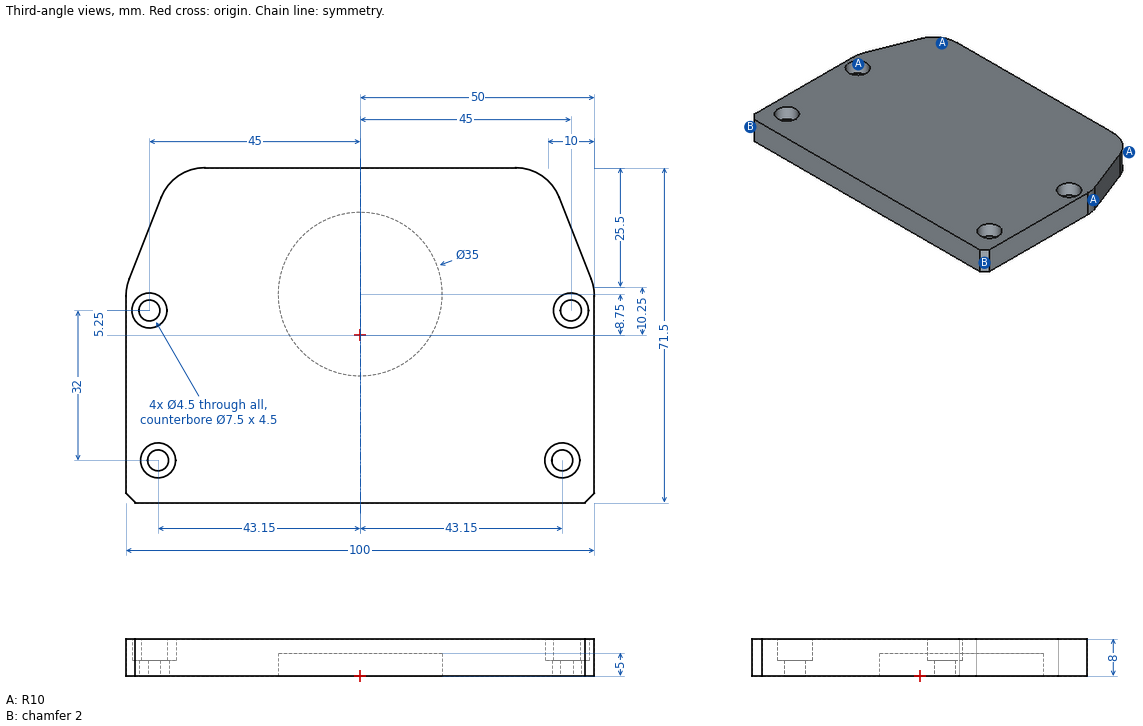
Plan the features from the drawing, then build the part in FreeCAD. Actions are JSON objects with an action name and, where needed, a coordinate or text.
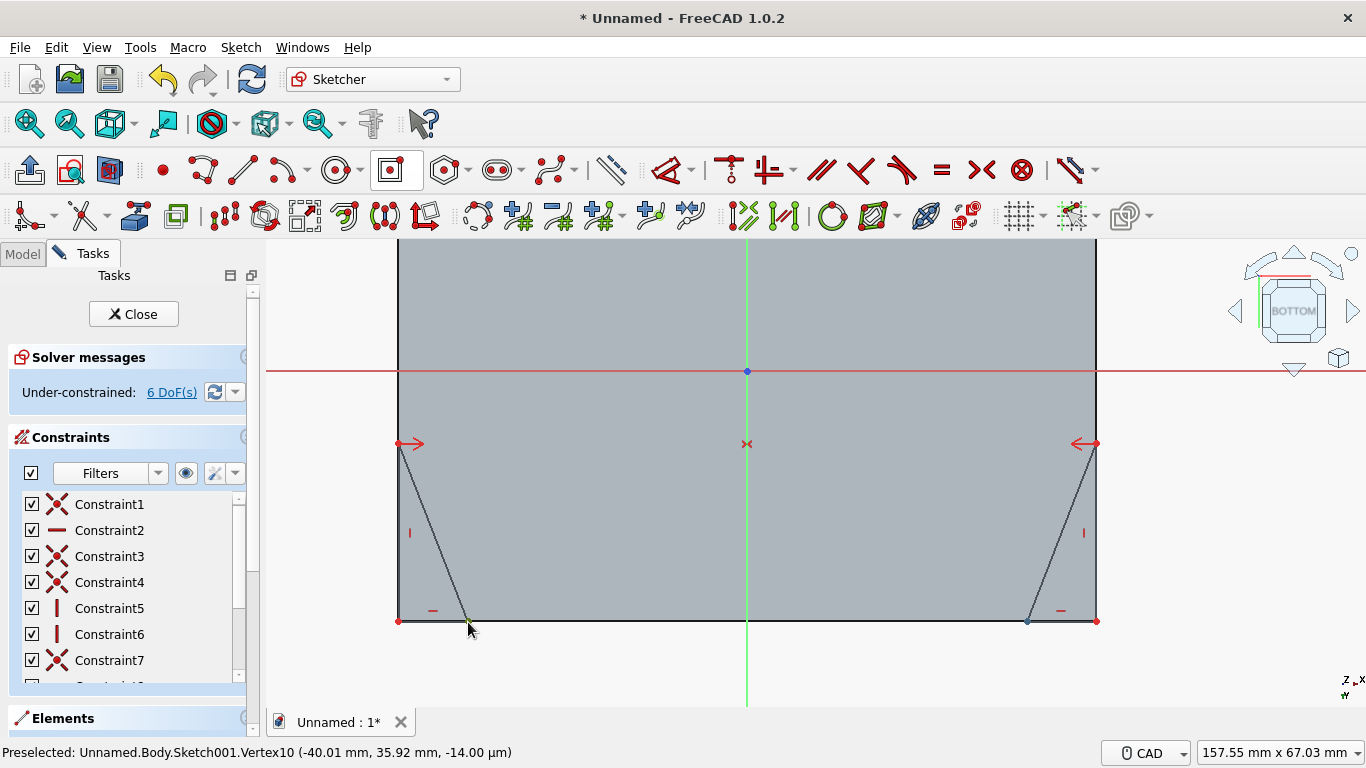
{"action": "left_click", "coordinate": [747, 650]}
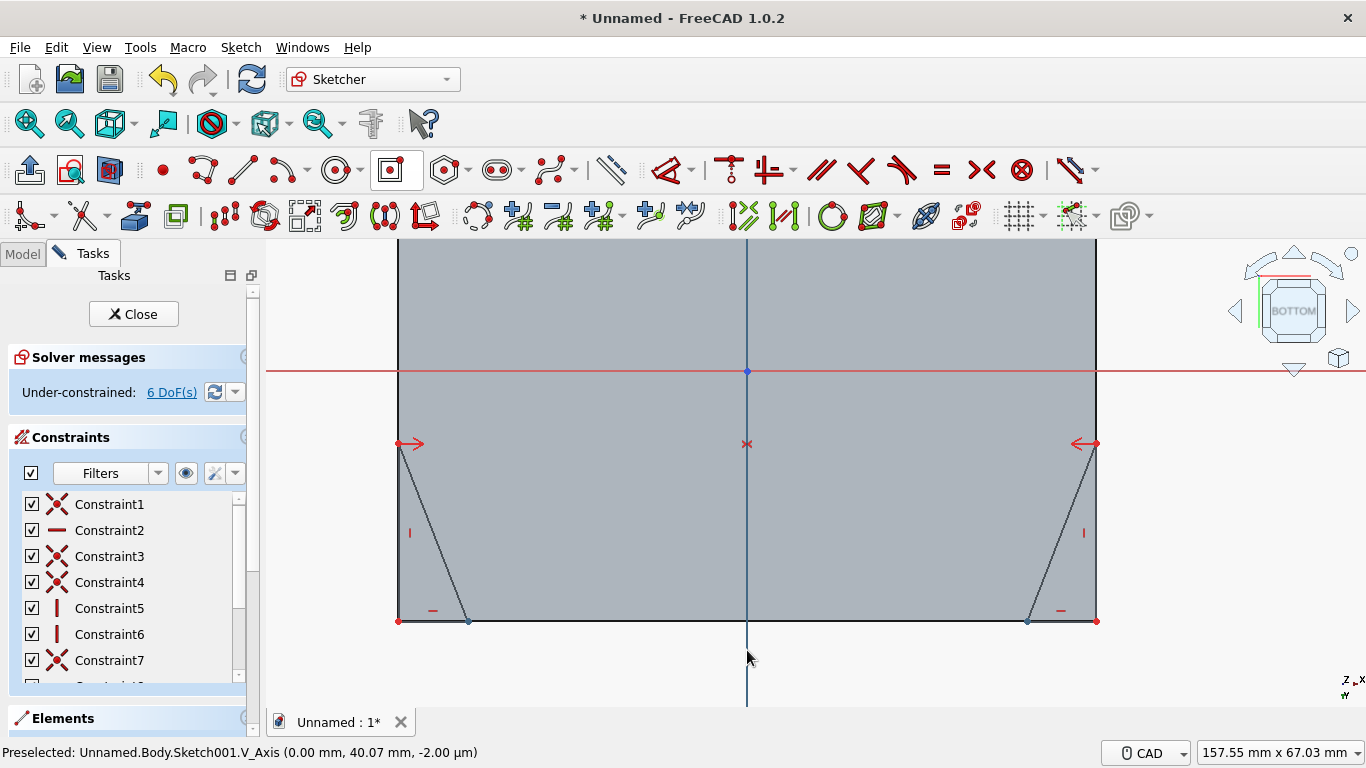
{"action": "left_click", "coordinate": [982, 170]}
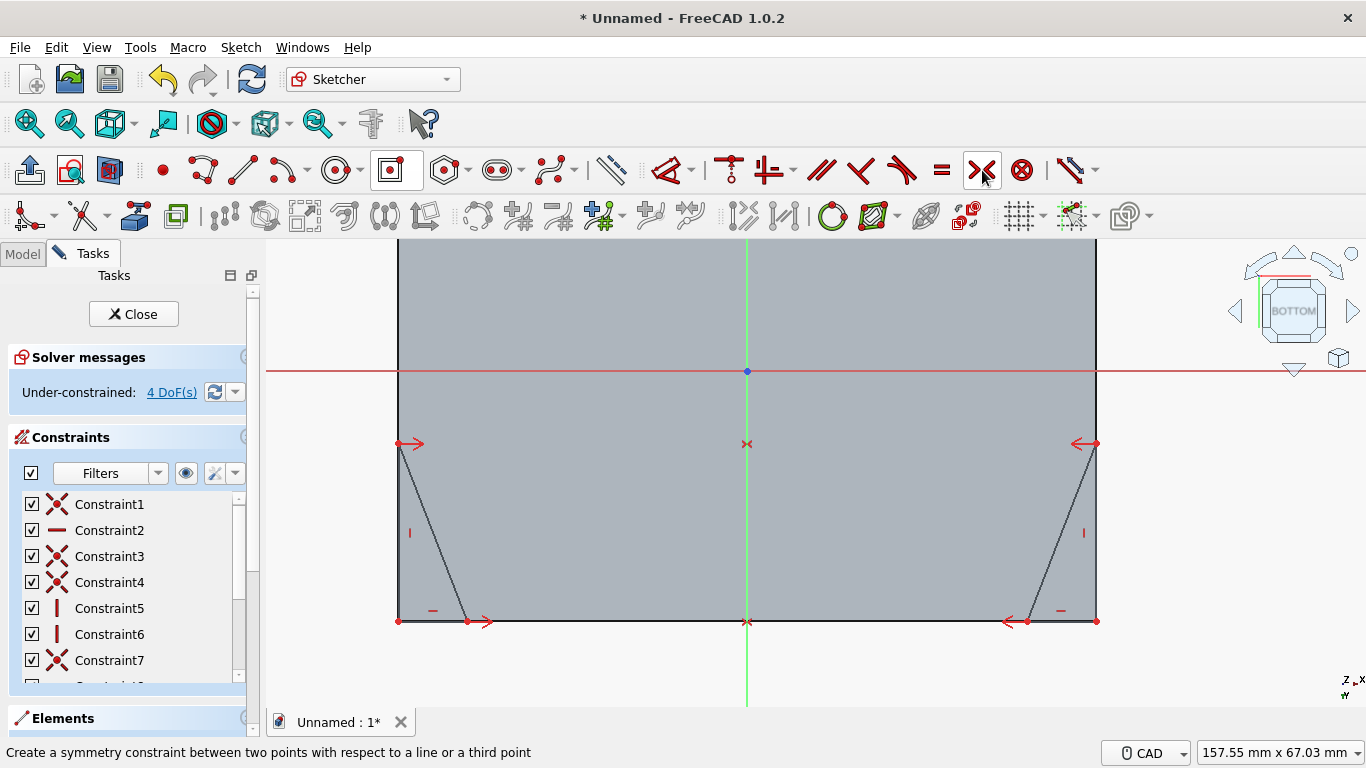
{"action": "left_click", "coordinate": [666, 170]}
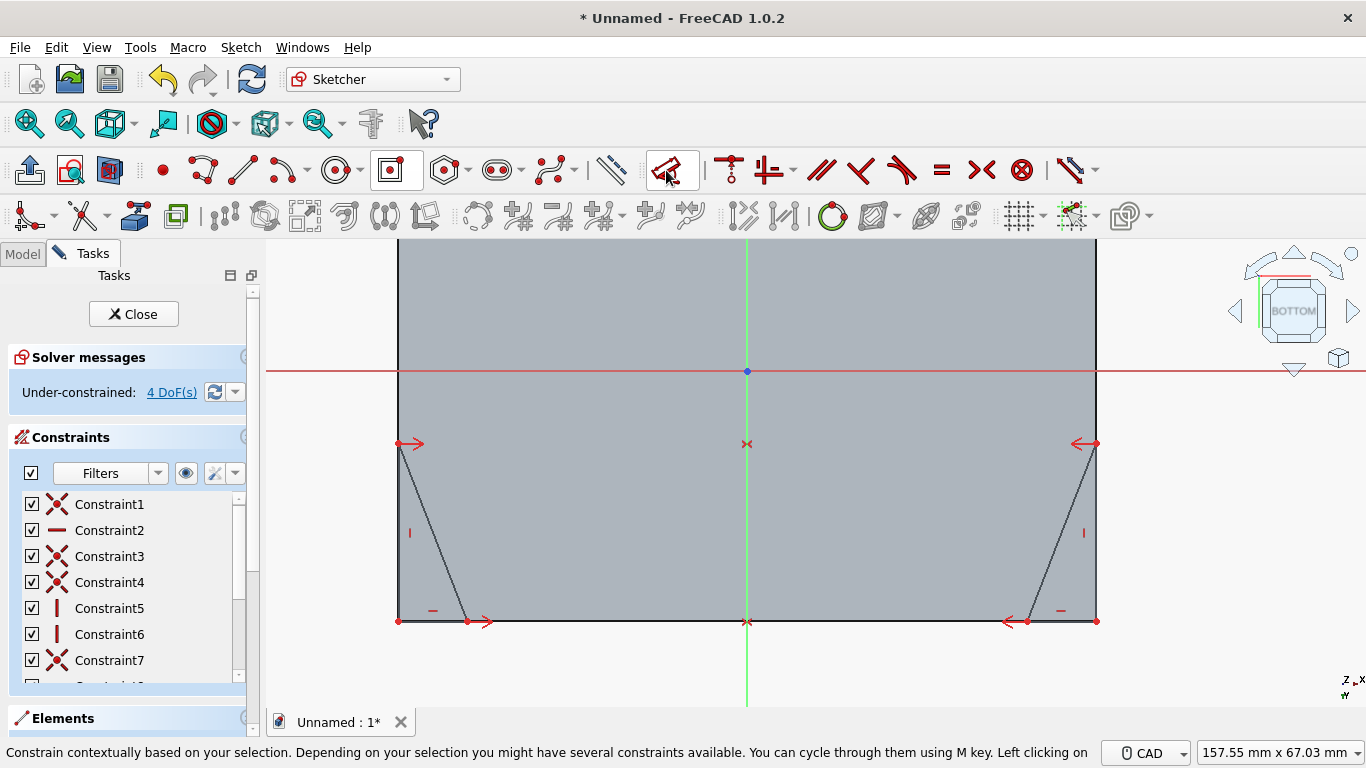
{"action": "left_click", "coordinate": [1048, 622]}
{"action": "left_click", "coordinate": [1062, 656]}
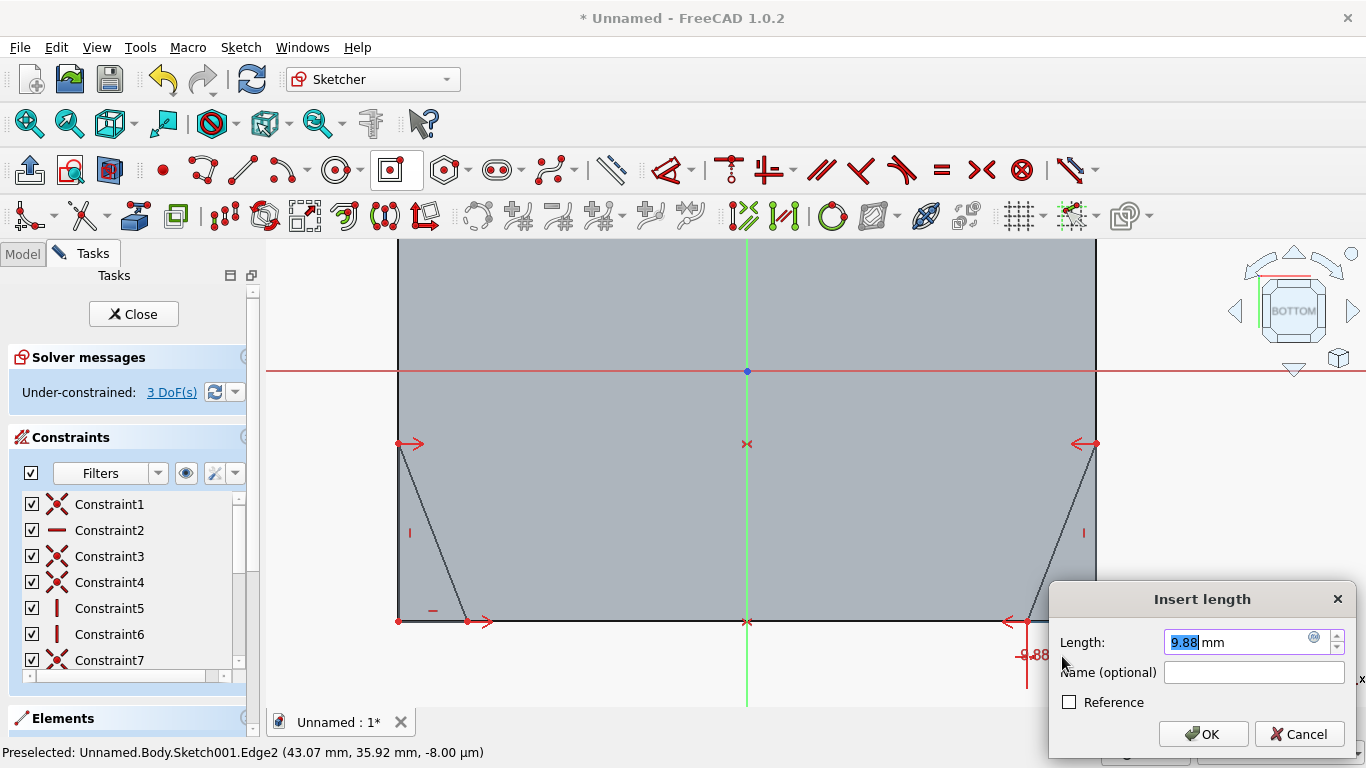
{"action": "type", "text": "10"}
{"action": "key", "text": "Return"}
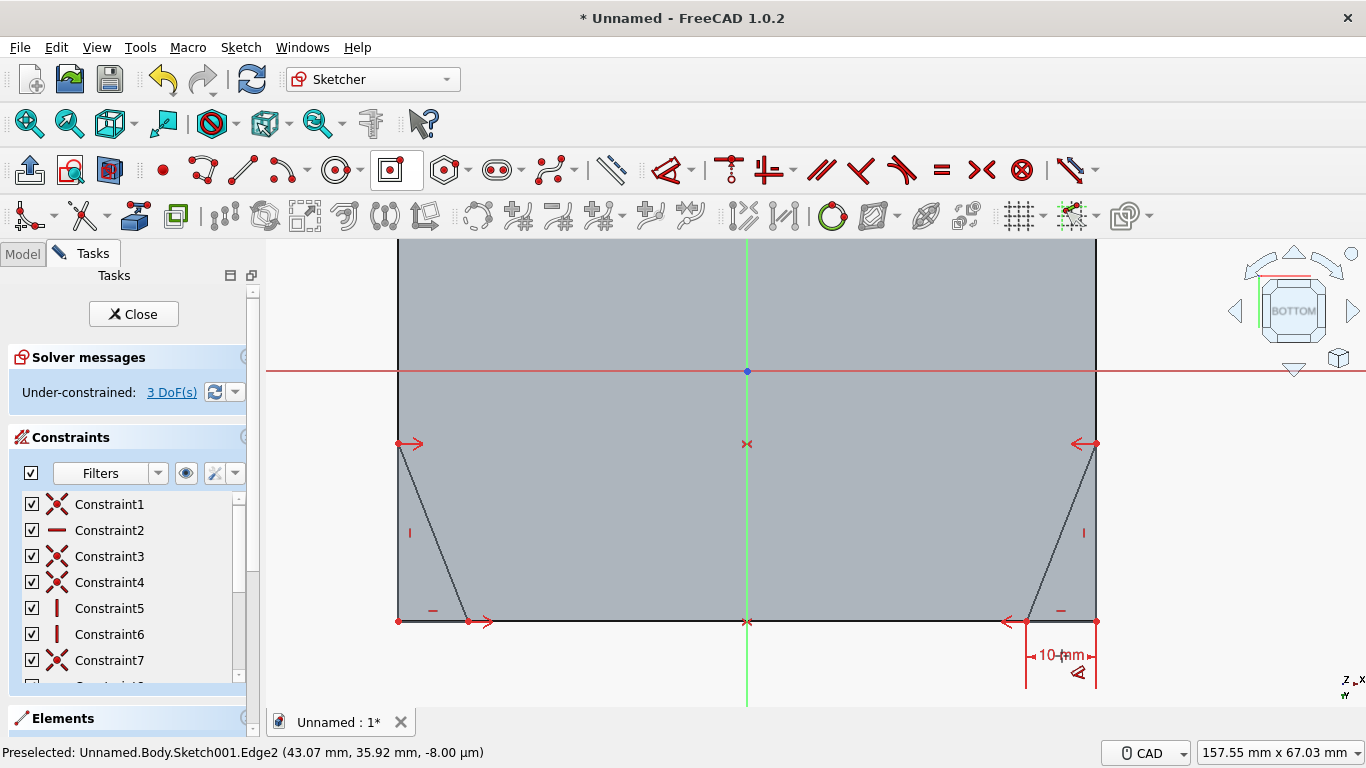
{"action": "left_click", "coordinate": [1096, 444]}
{"action": "left_click", "coordinate": [922, 337]}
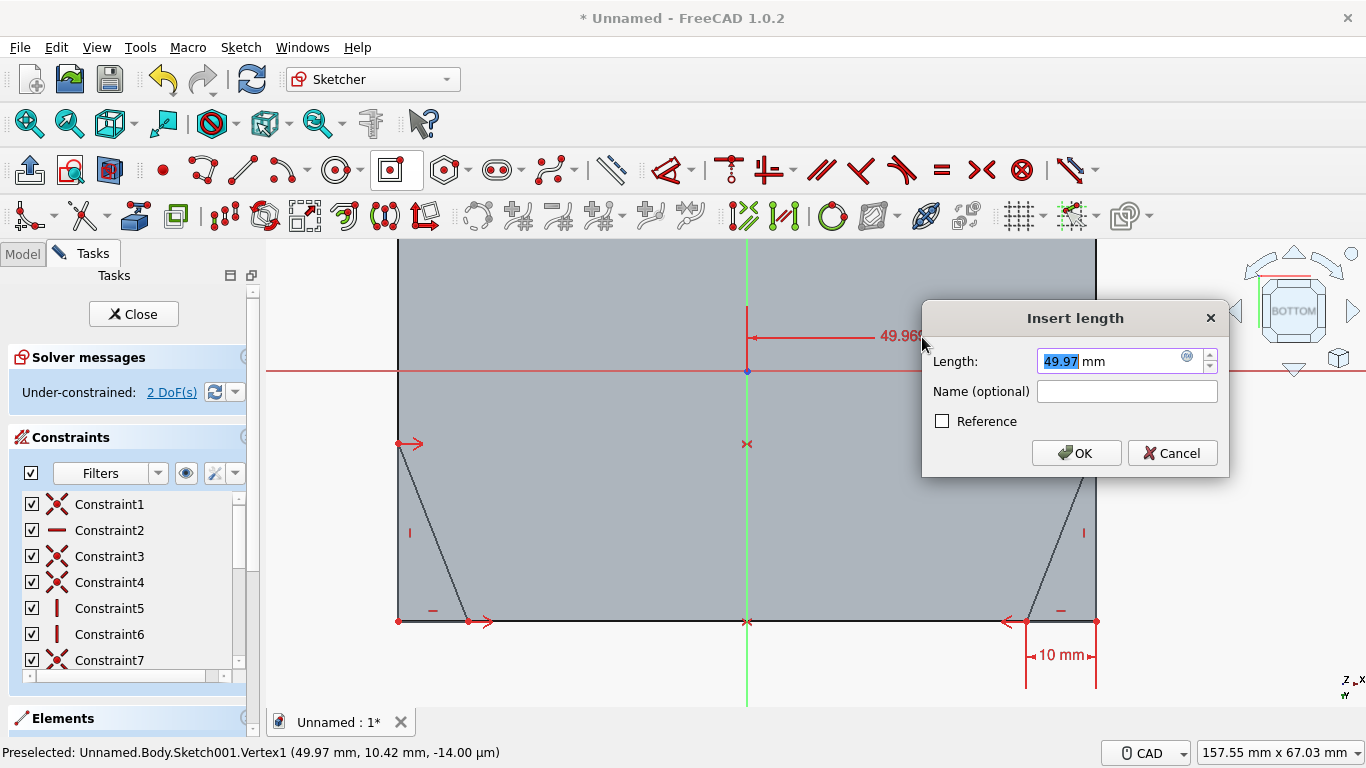
{"action": "type", "text": "50"}
{"action": "key", "text": "Return"}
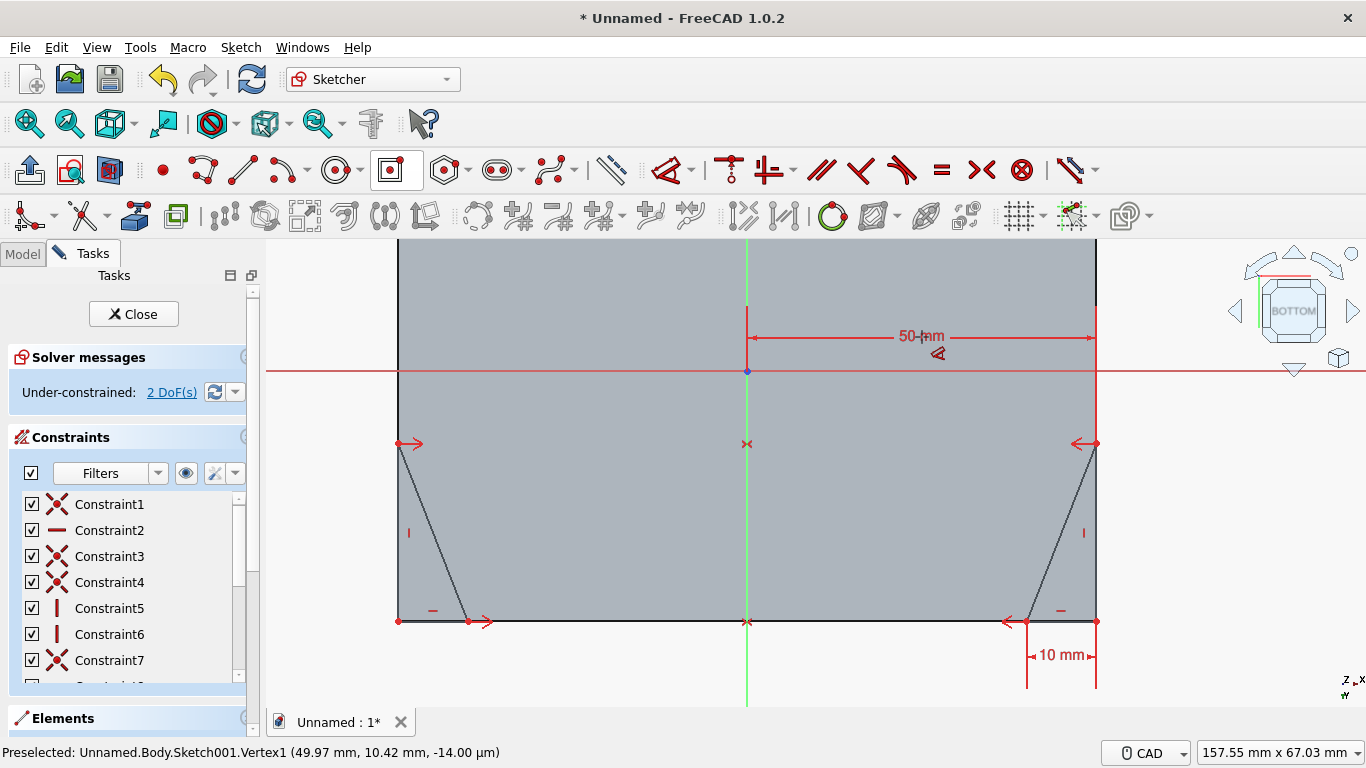
{"action": "left_click", "coordinate": [1096, 569]}
{"action": "left_click", "coordinate": [1130, 533]}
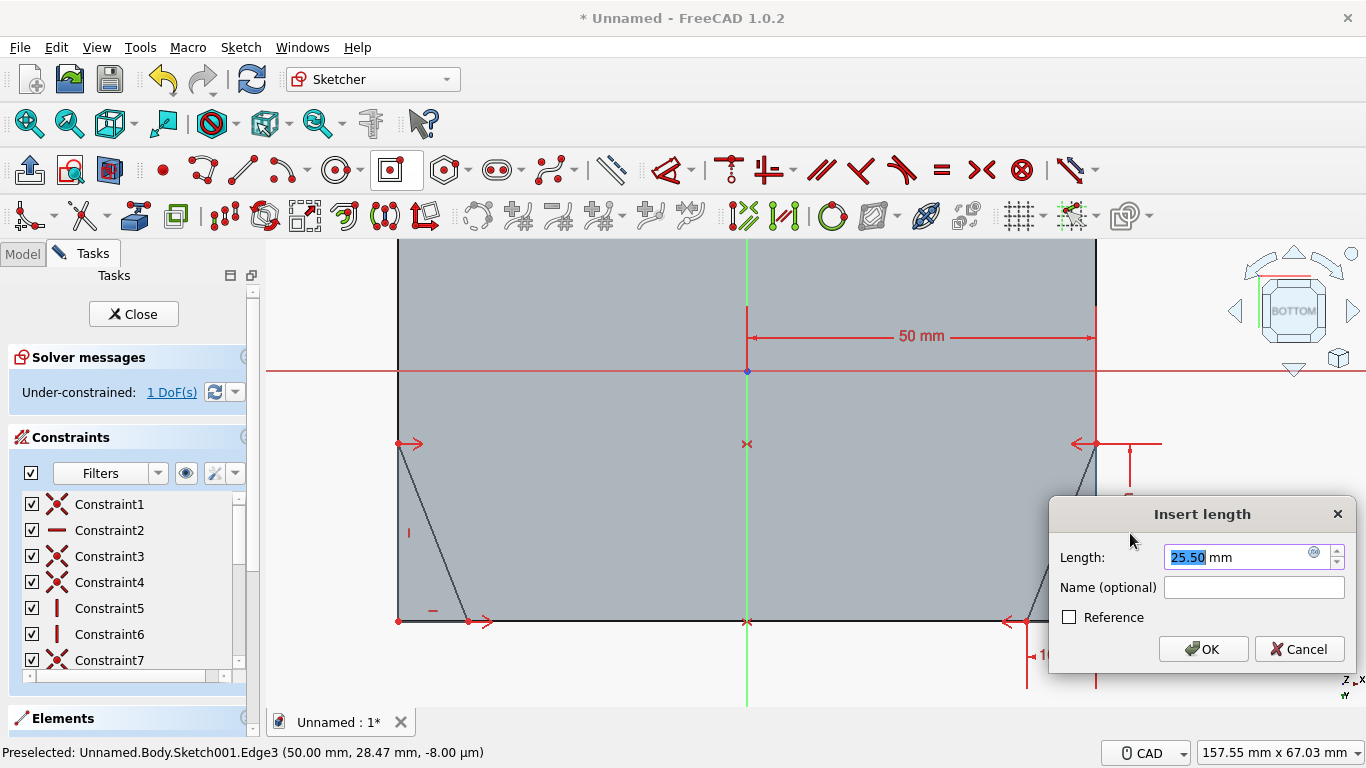
{"action": "type", "text": "25.5"}
{"action": "key", "text": "Return"}